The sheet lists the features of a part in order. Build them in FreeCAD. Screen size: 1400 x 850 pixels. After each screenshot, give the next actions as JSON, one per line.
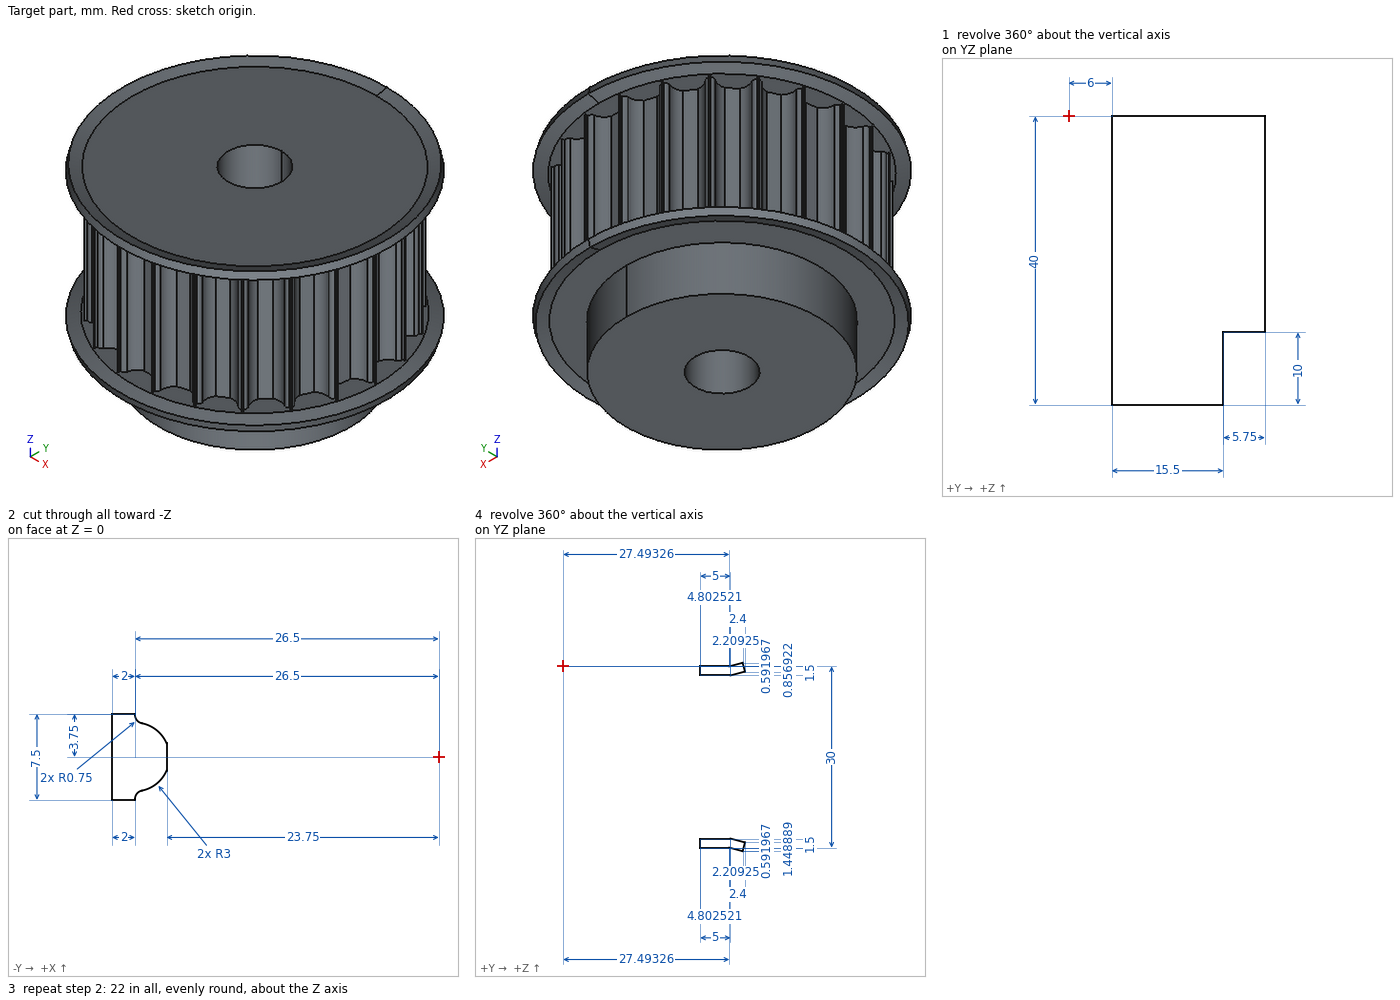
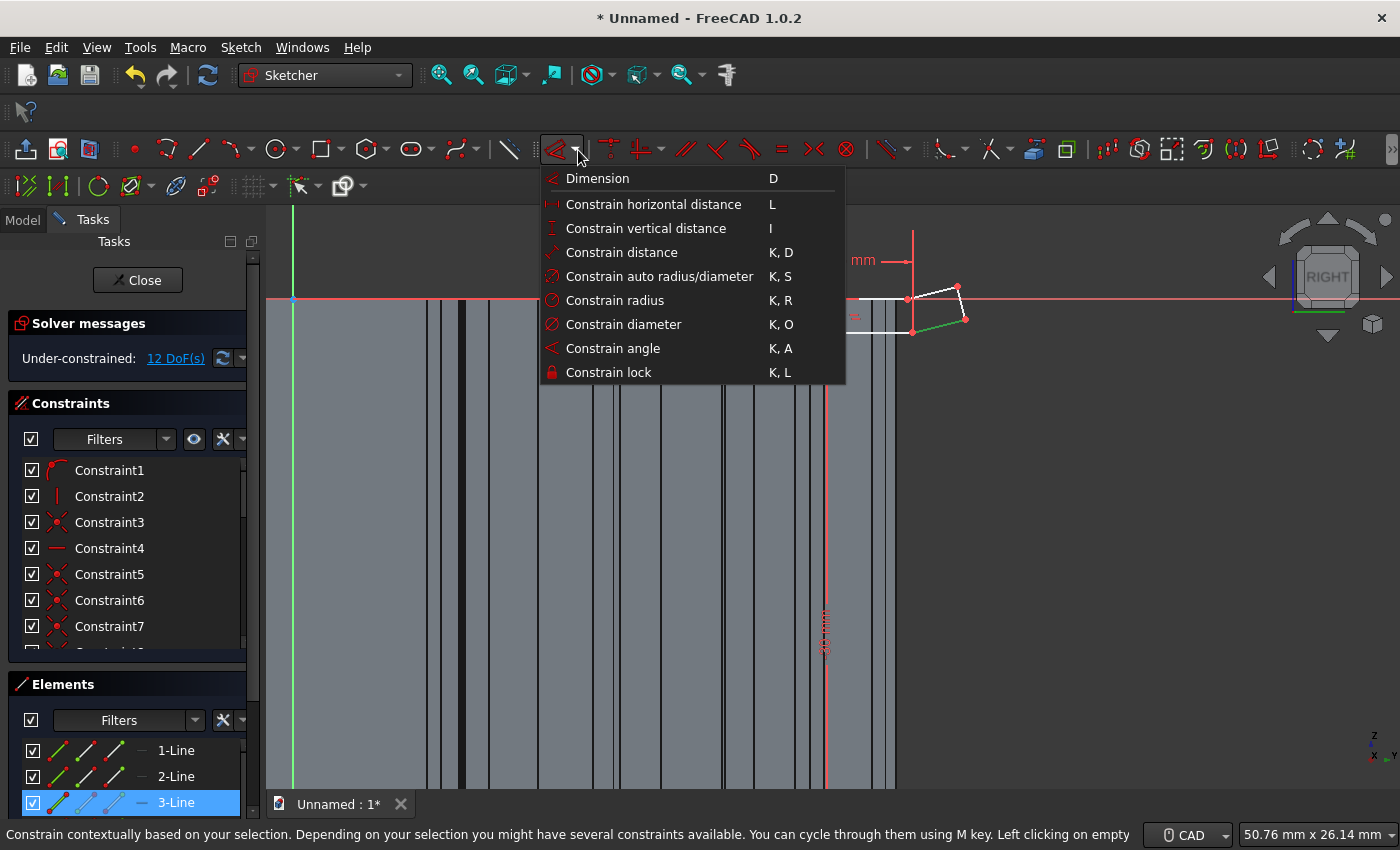
{"action": "left_click", "coordinate": [693, 204]}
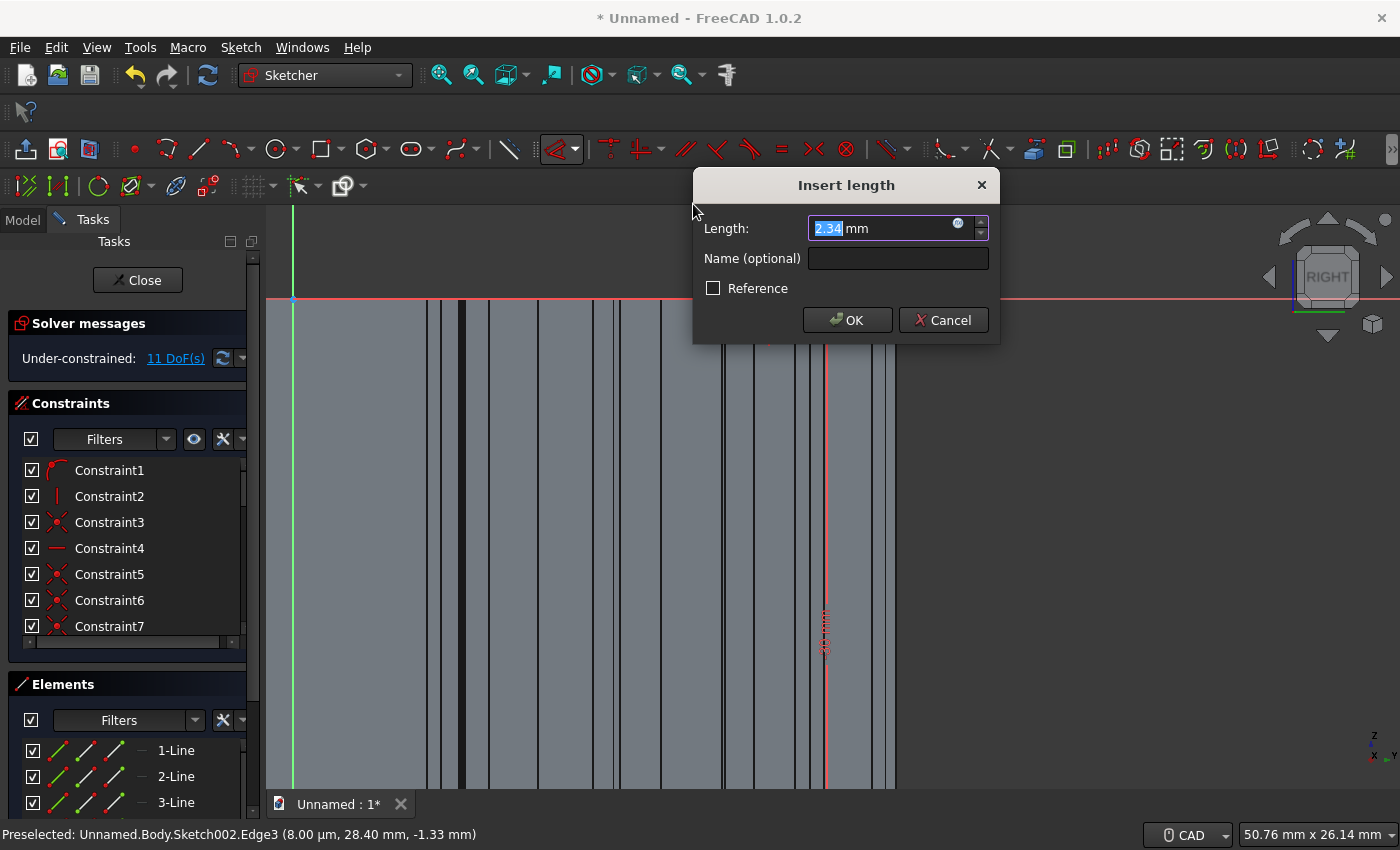
{"action": "type", "text": "2.4"}
{"action": "key", "text": "Return"}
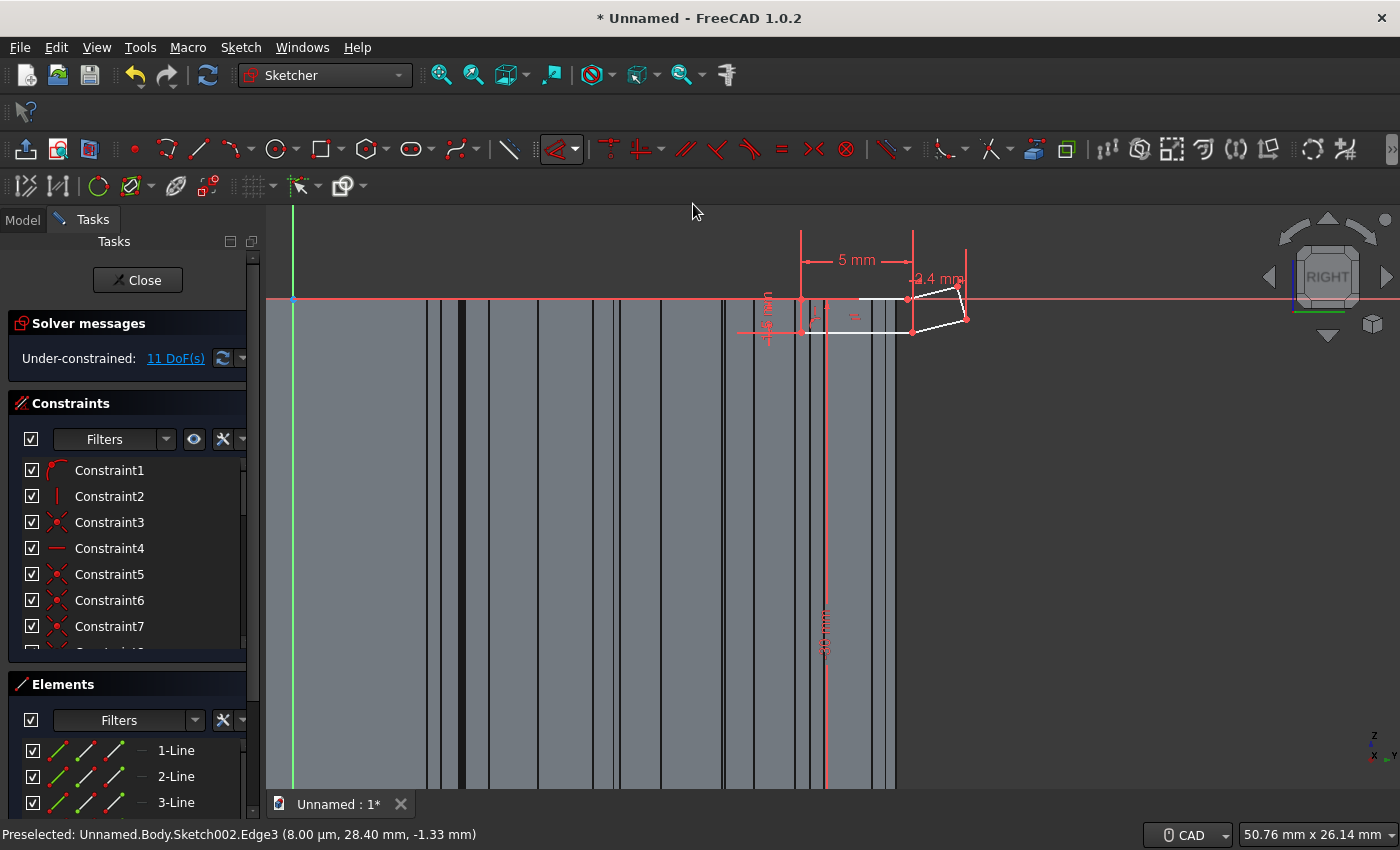
{"action": "scroll", "coordinate": [929, 330], "scroll_direction": "down", "scroll_amount": 3}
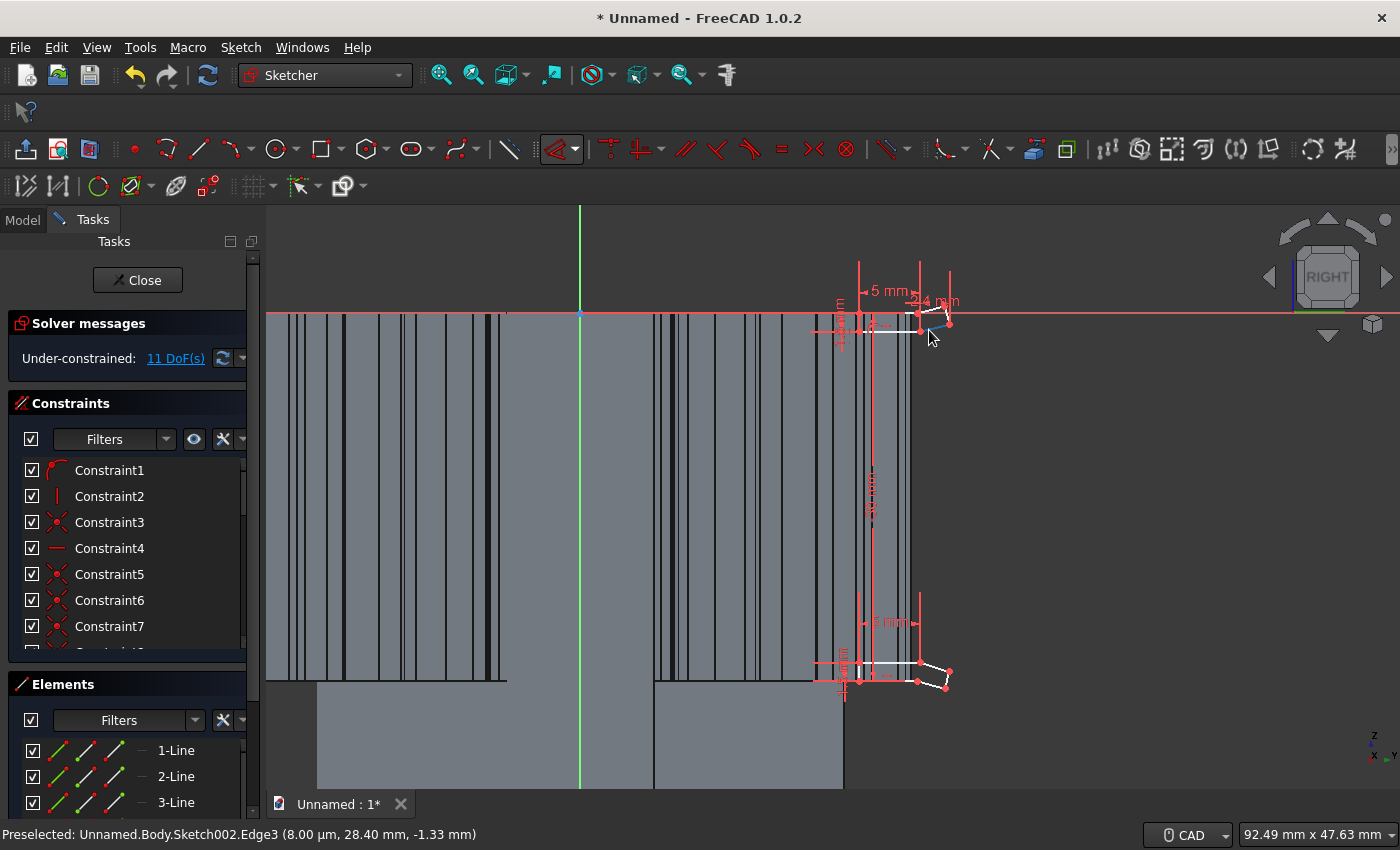
{"action": "scroll", "coordinate": [940, 669], "scroll_direction": "up", "scroll_amount": 3}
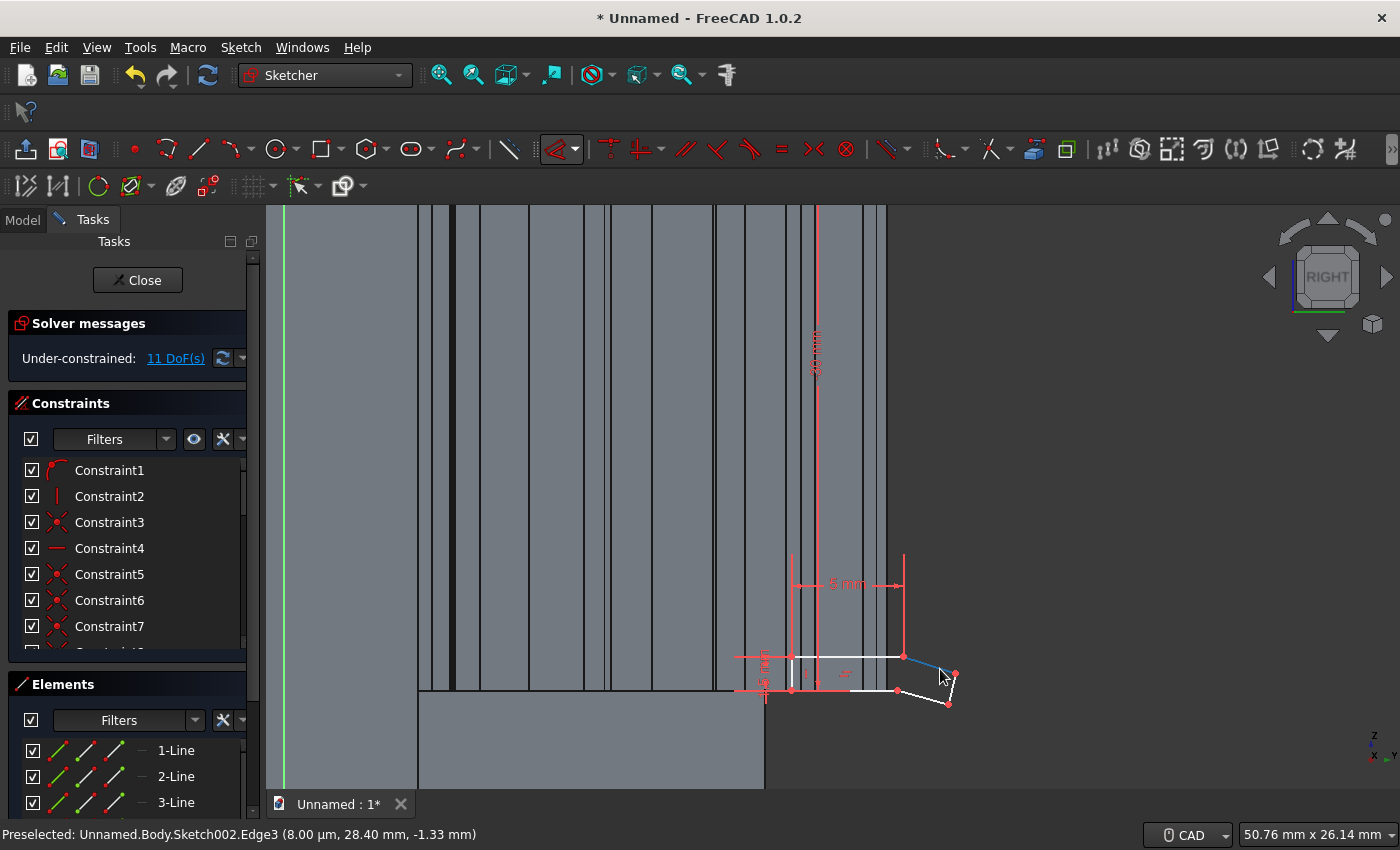
{"action": "left_click", "coordinate": [940, 669]}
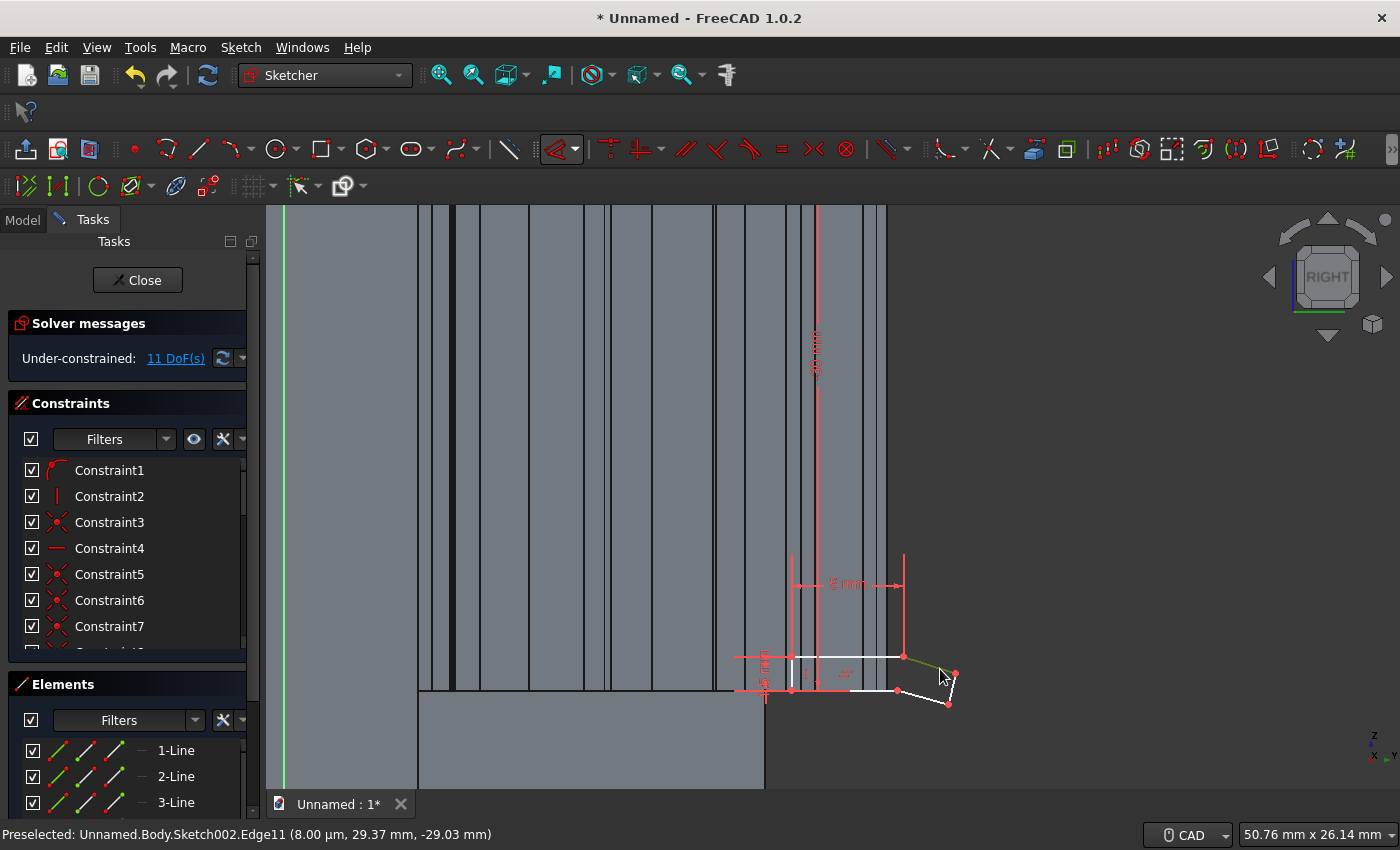
{"action": "left_click", "coordinate": [578, 150]}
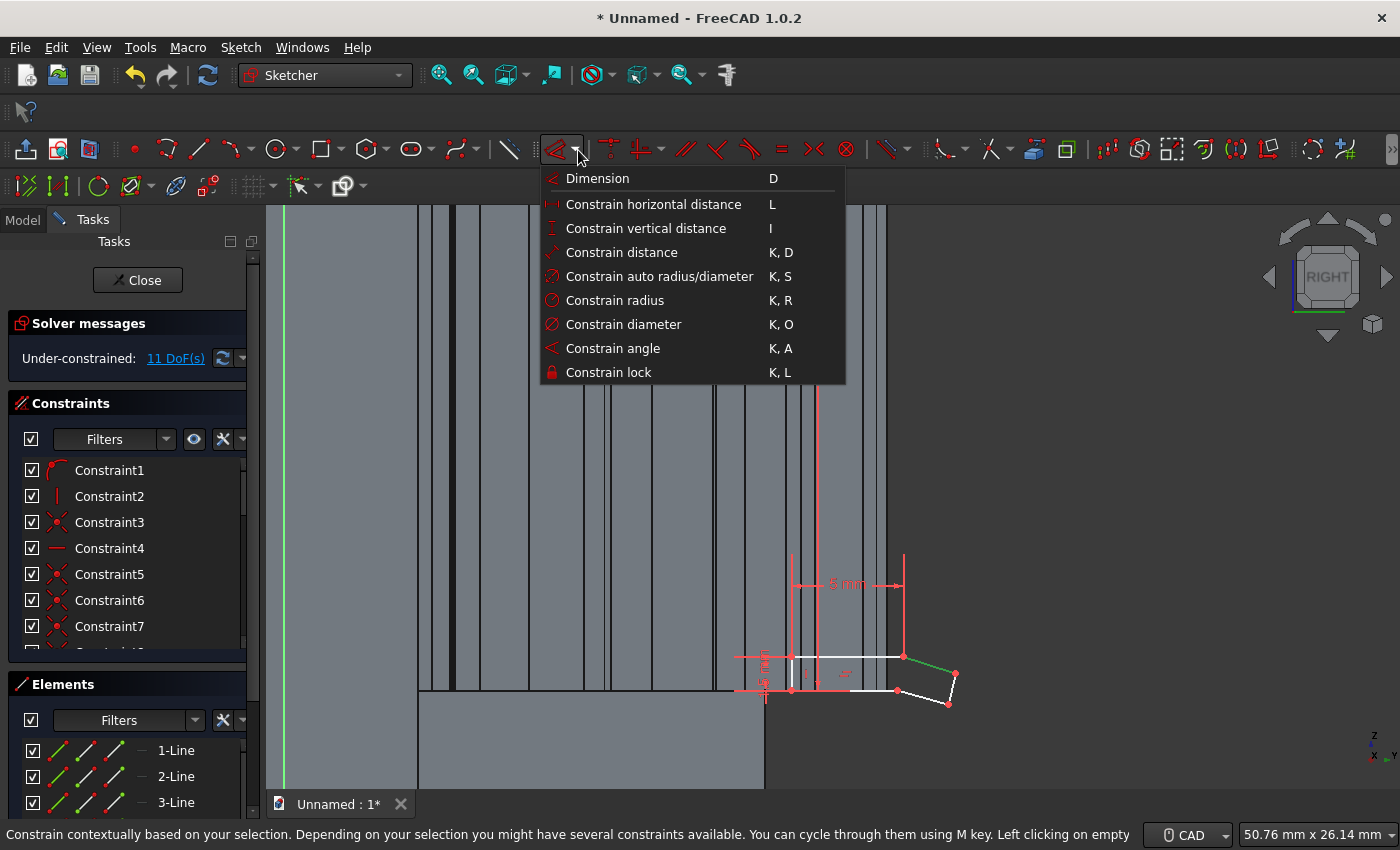
{"action": "left_click", "coordinate": [693, 204]}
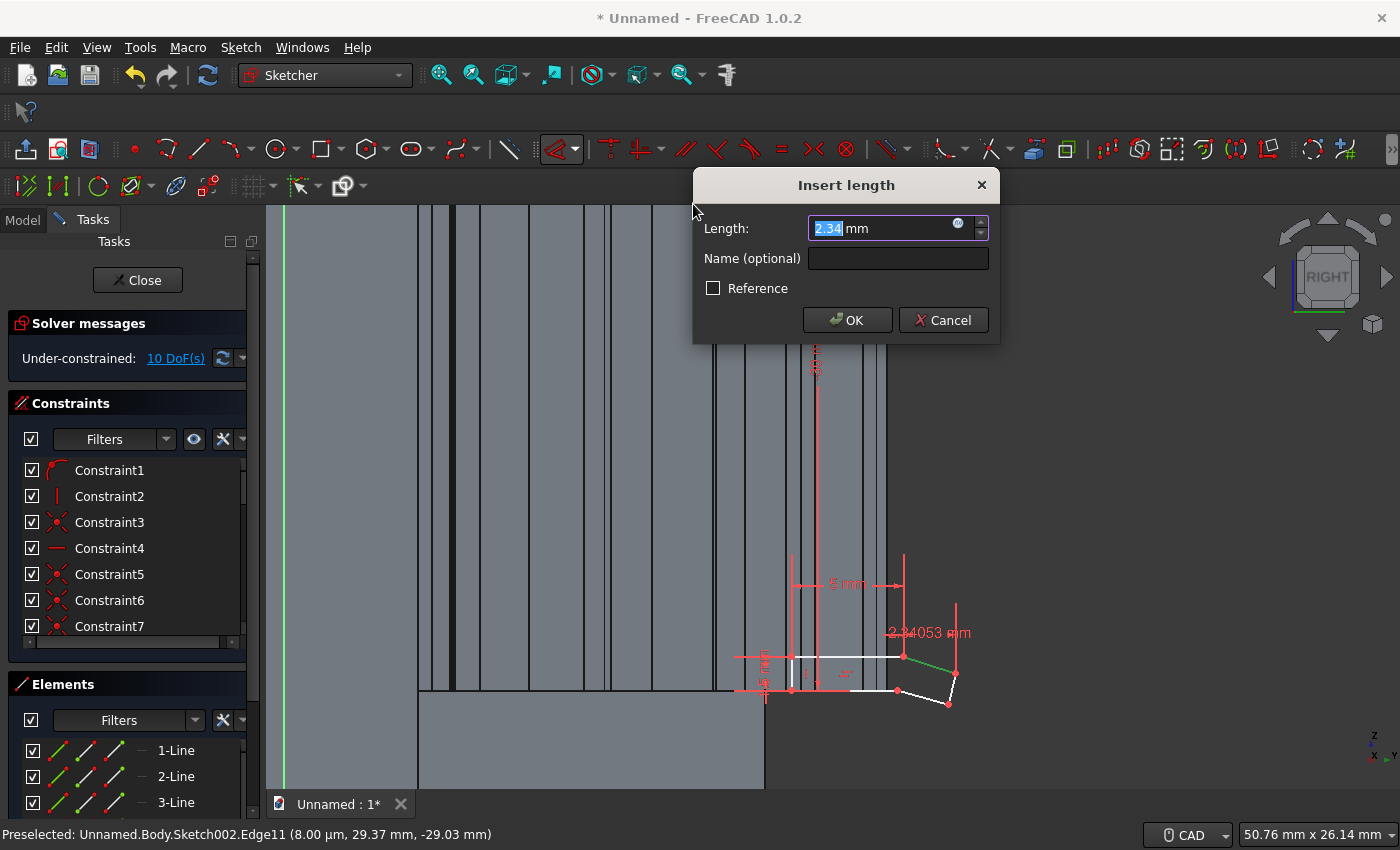
{"action": "type", "text": "2.4"}
{"action": "key", "text": "Return"}